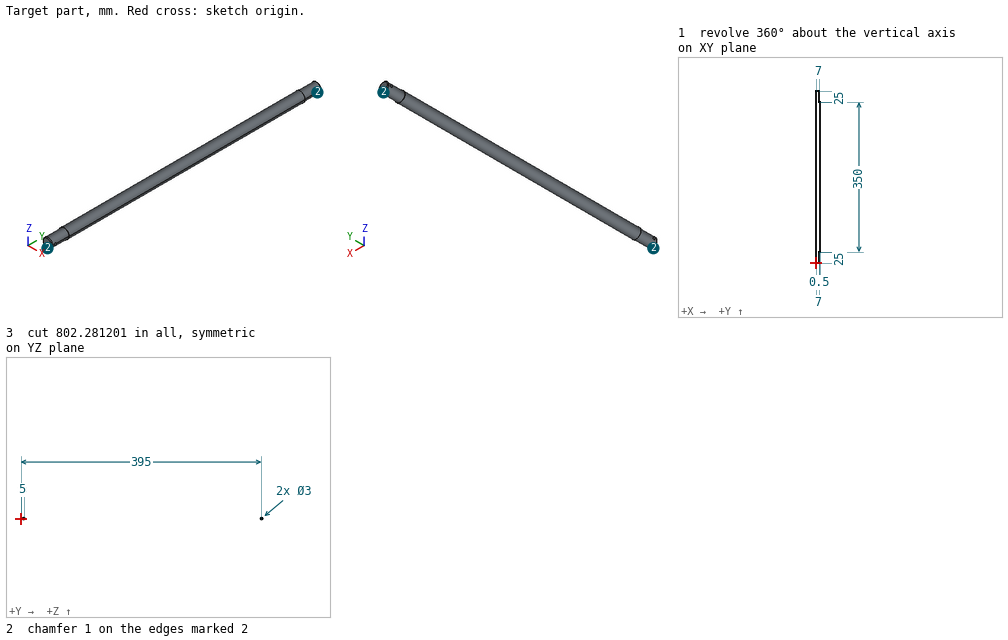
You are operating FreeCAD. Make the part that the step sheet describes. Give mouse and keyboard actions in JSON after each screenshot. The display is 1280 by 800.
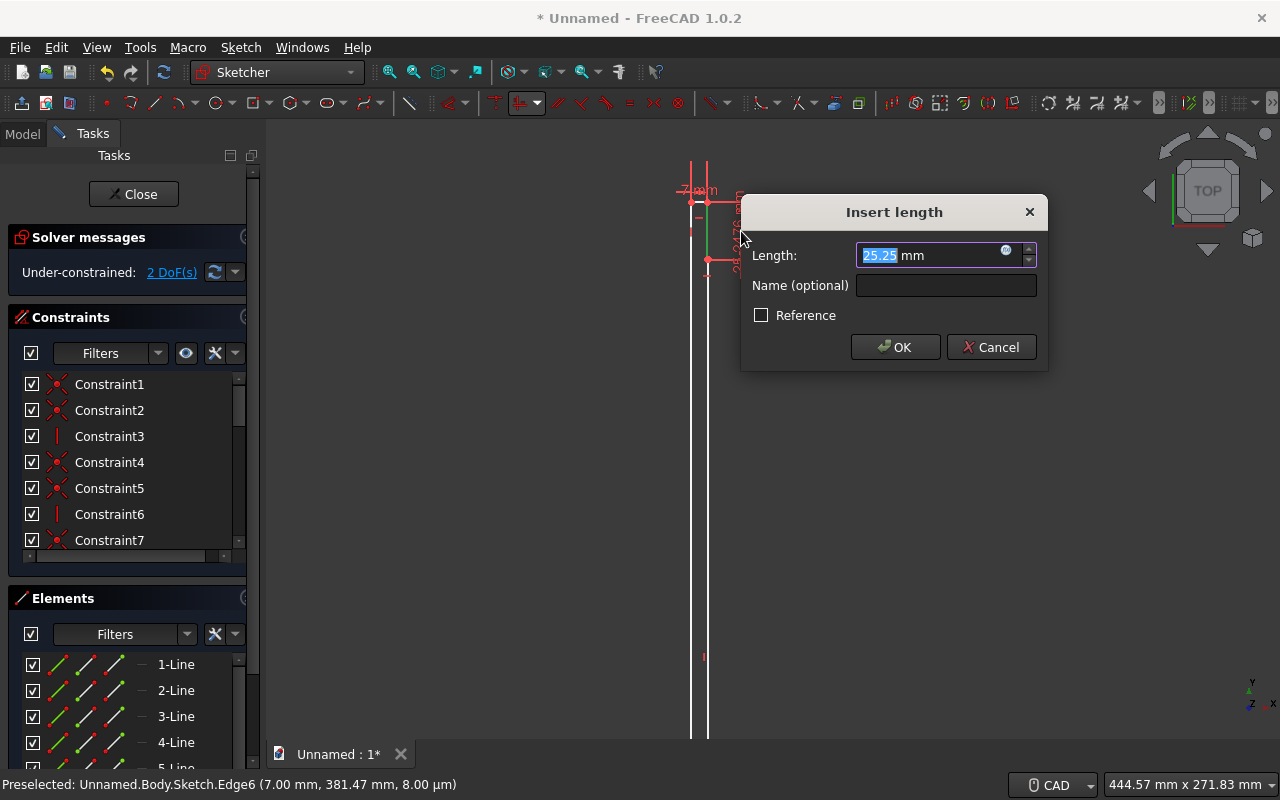
{"action": "type", "text": "25"}
{"action": "key", "text": "Return"}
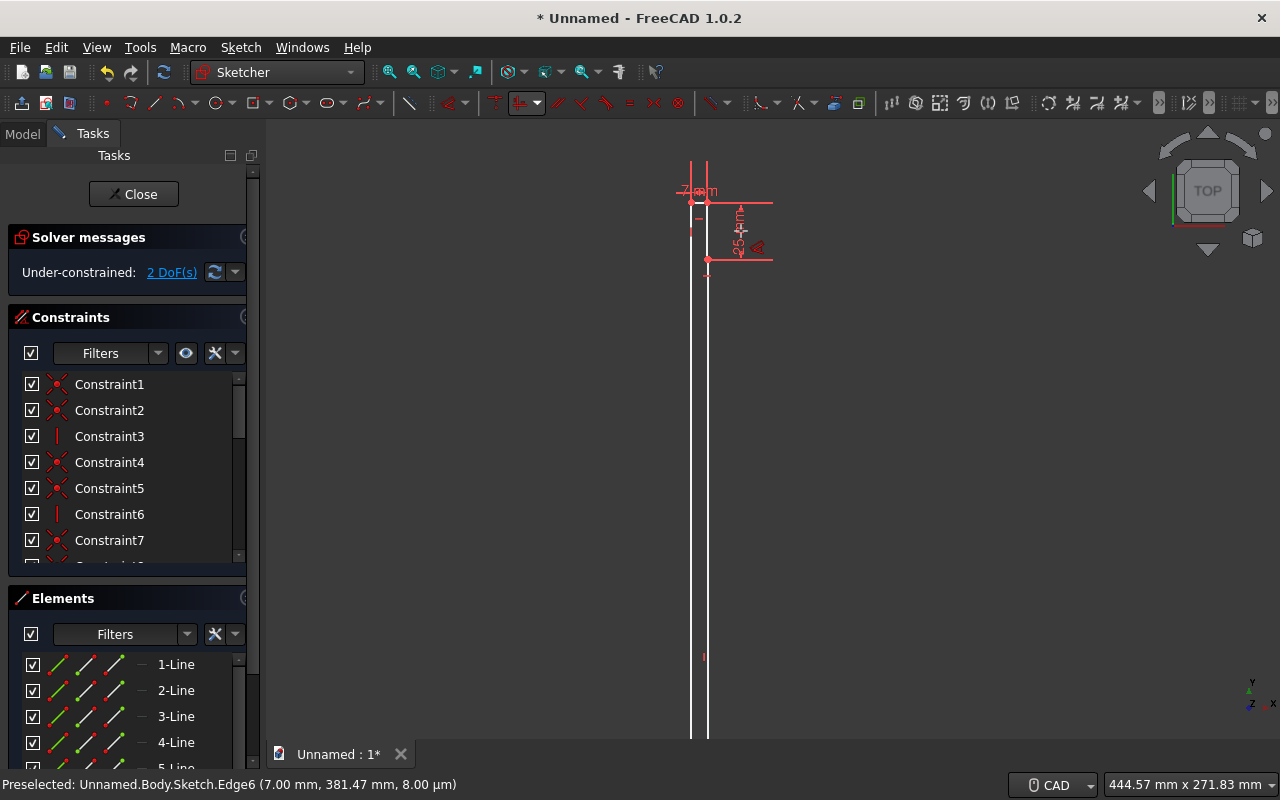
{"action": "scroll", "coordinate": [708, 242], "scroll_direction": "down", "scroll_amount": 4}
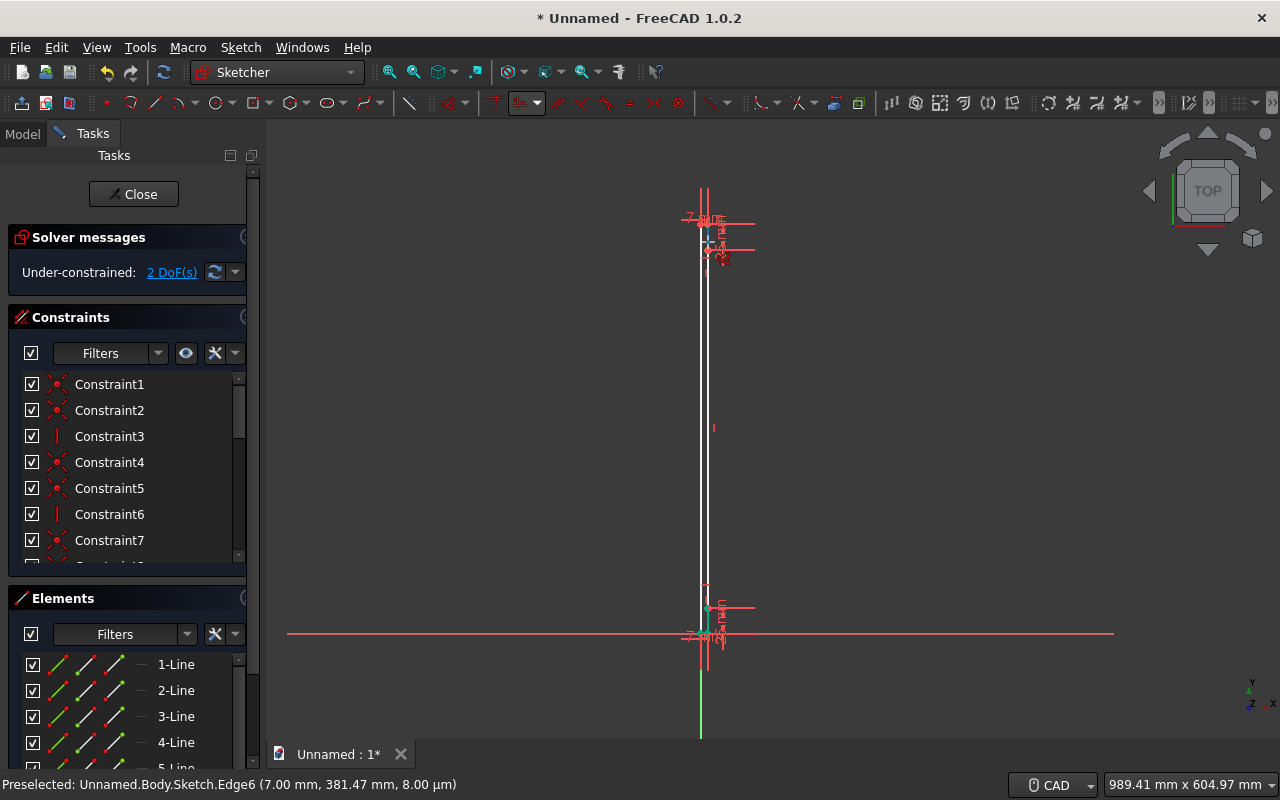
{"action": "scroll", "coordinate": [708, 608], "scroll_direction": "up", "scroll_amount": 22}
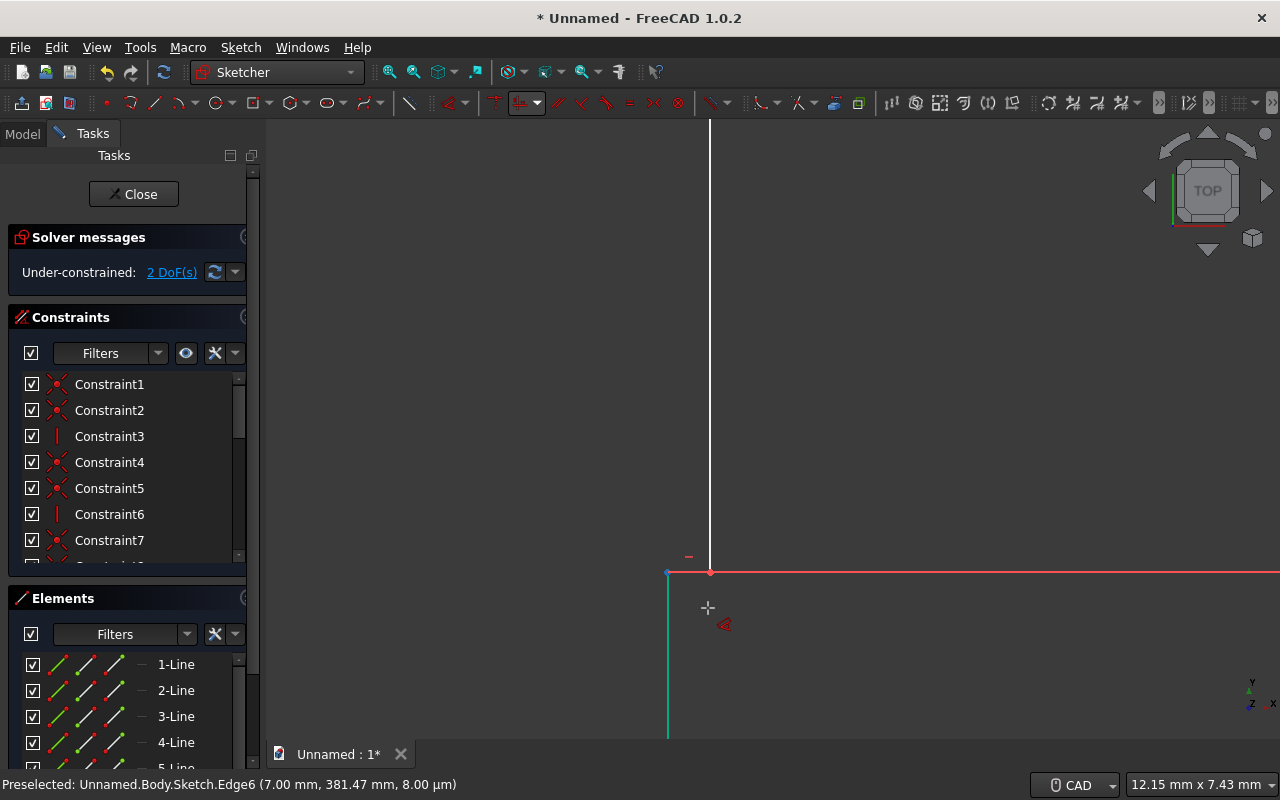
{"action": "left_click", "coordinate": [689, 572]}
{"action": "left_click", "coordinate": [689, 606]}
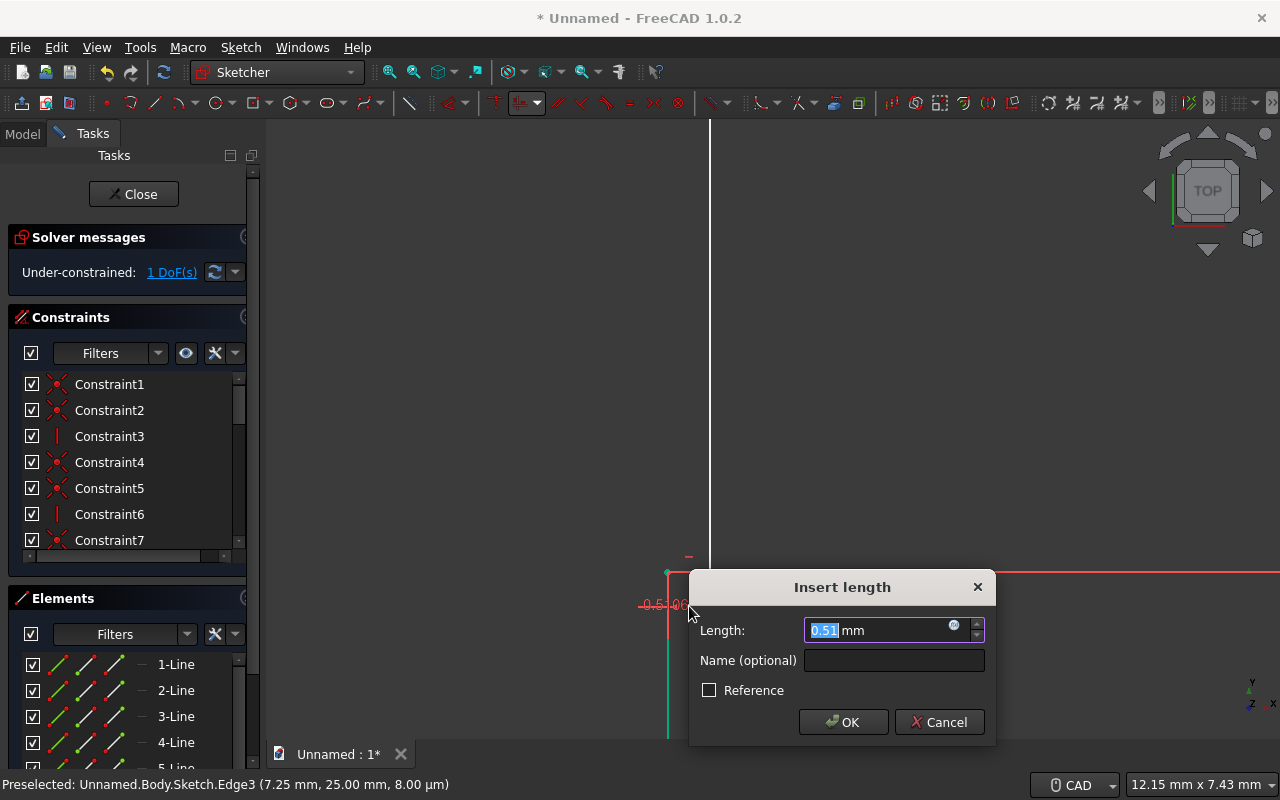
{"action": "type", "text": "0.5"}
{"action": "key", "text": "Return"}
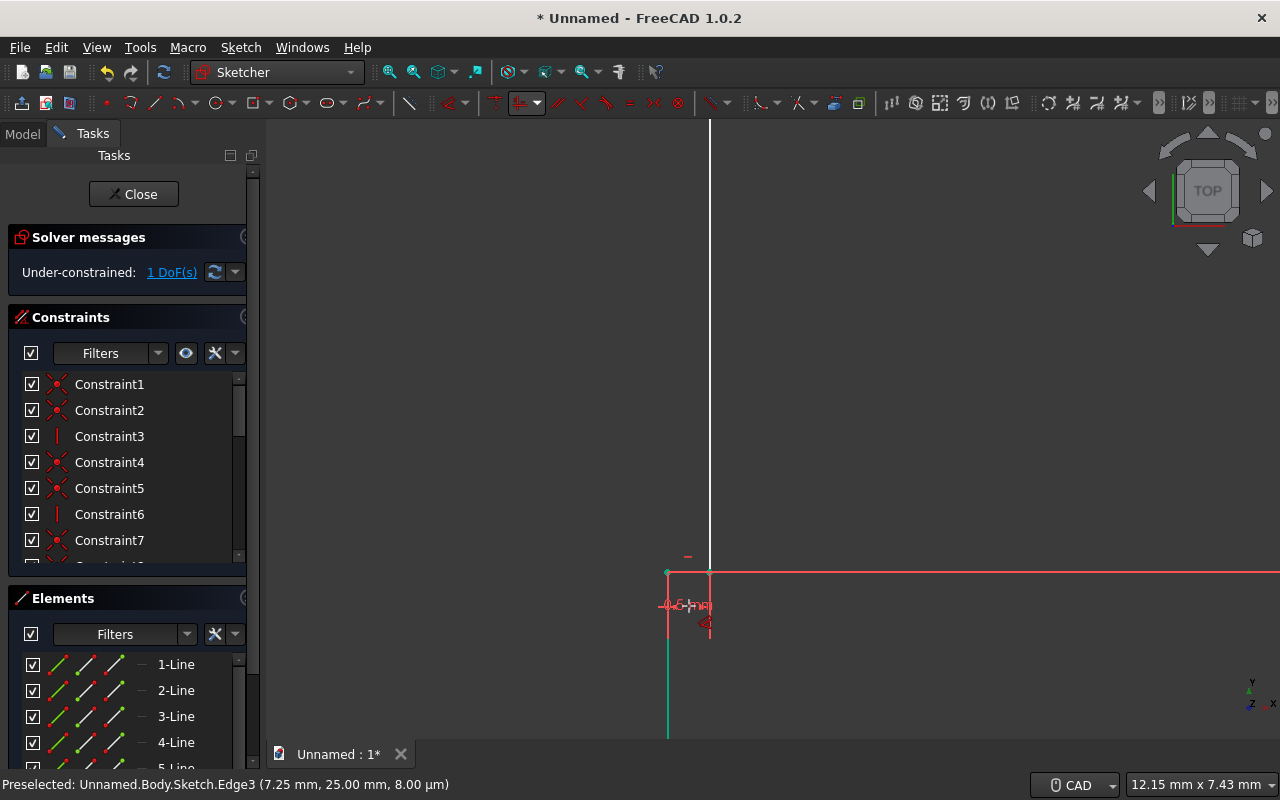
{"action": "scroll", "coordinate": [704, 429], "scroll_direction": "down", "scroll_amount": 15}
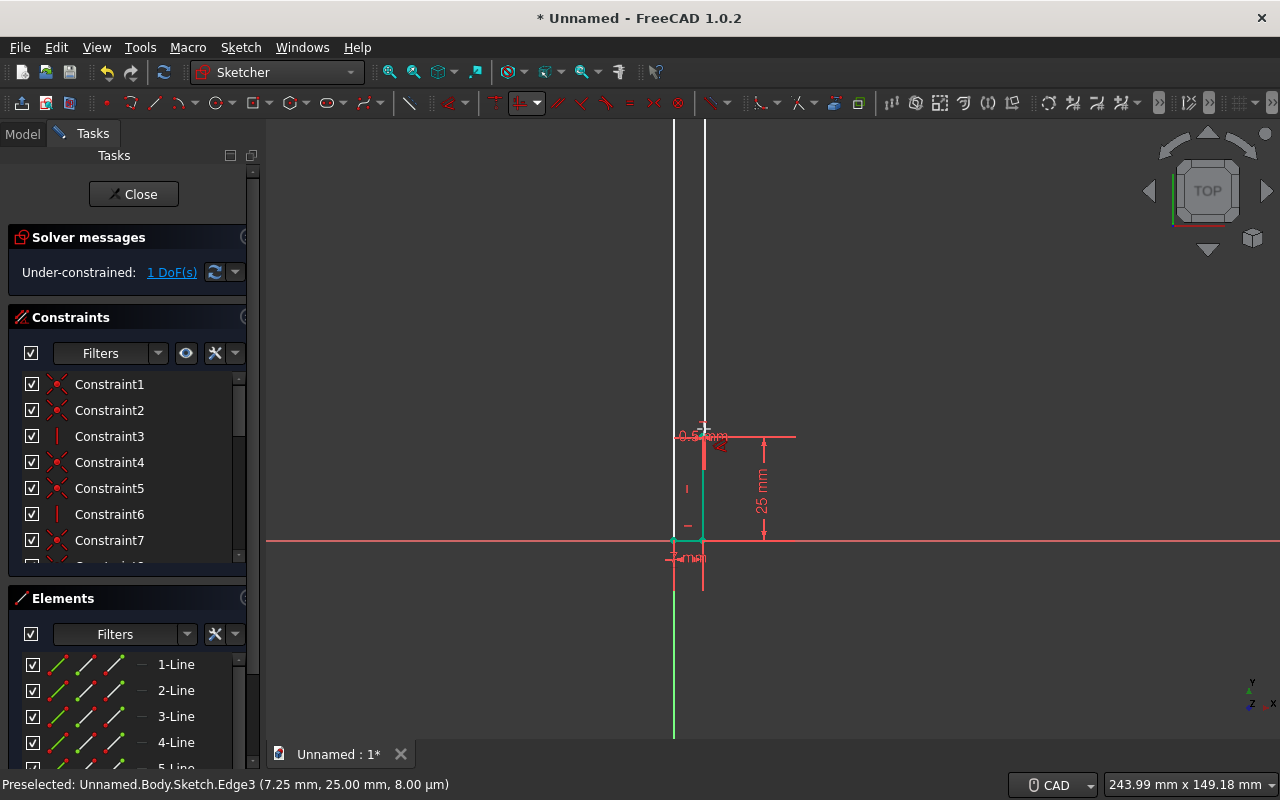
{"action": "scroll", "coordinate": [710, 665], "scroll_direction": "down", "scroll_amount": 7}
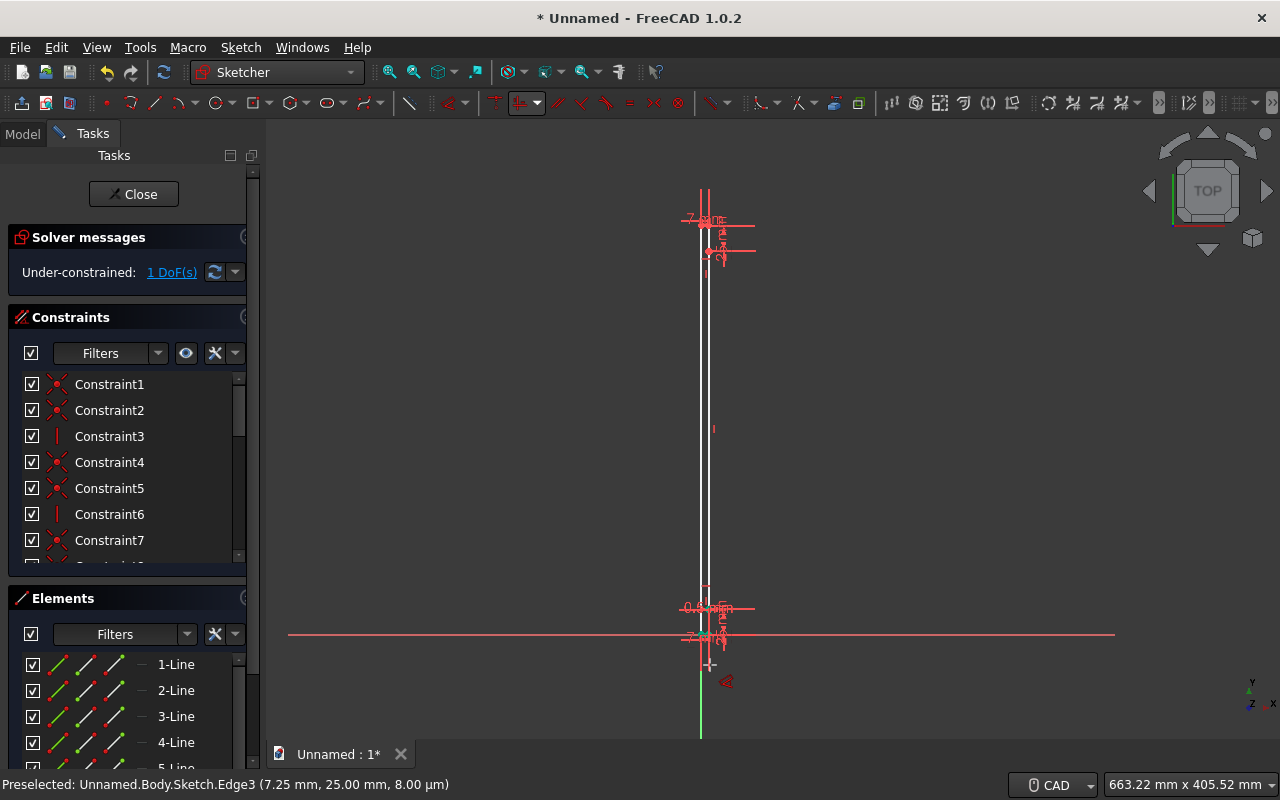
{"action": "scroll", "coordinate": [709, 502], "scroll_direction": "up", "scroll_amount": 3}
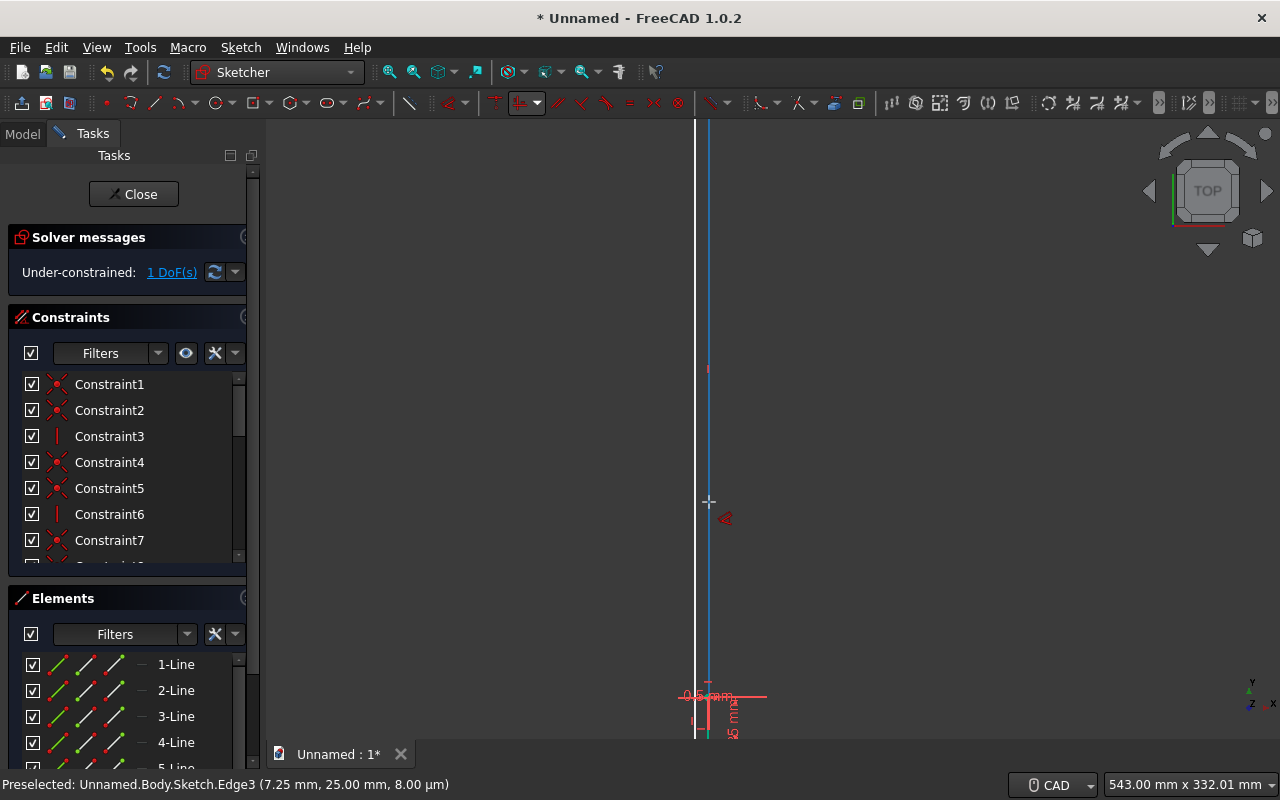
{"action": "left_click", "coordinate": [709, 501]}
{"action": "left_click", "coordinate": [743, 422]}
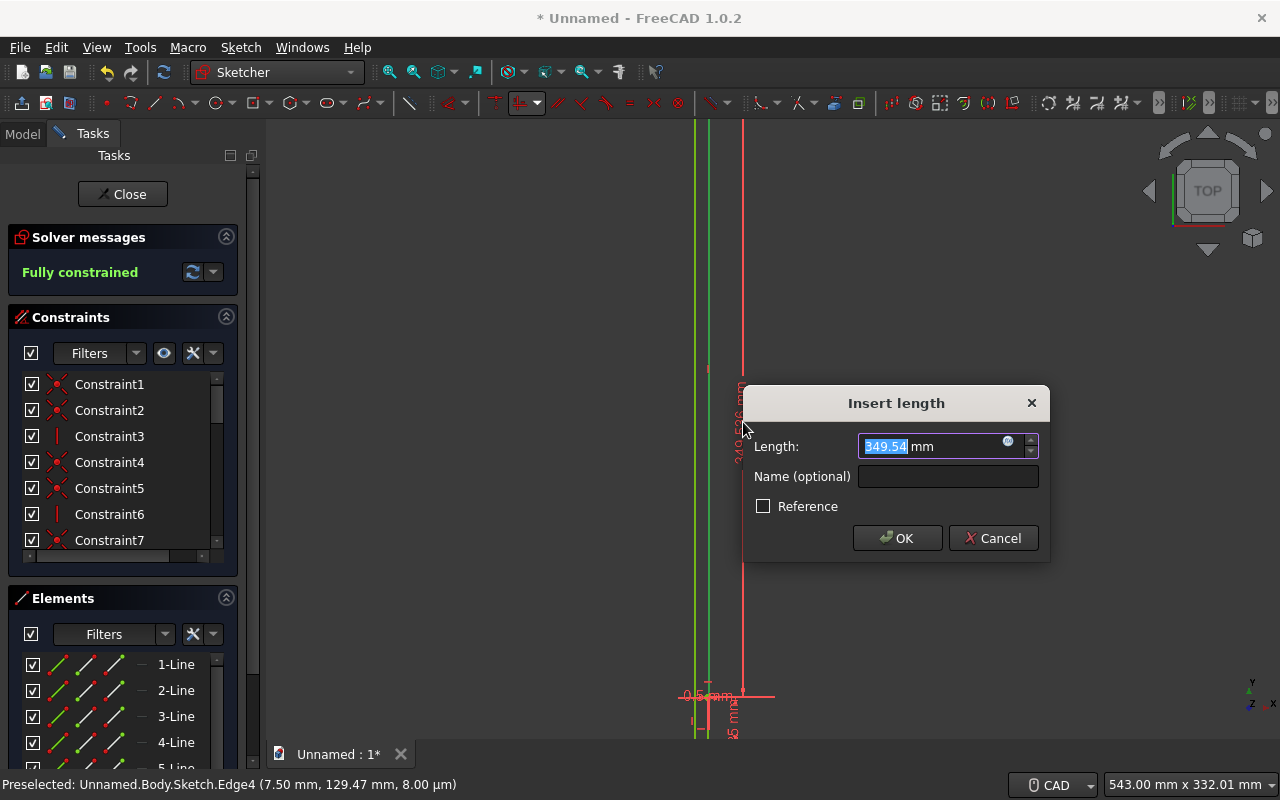
{"action": "type", "text": "350"}
{"action": "key", "text": "Return"}
{"action": "key", "text": "Escape"}